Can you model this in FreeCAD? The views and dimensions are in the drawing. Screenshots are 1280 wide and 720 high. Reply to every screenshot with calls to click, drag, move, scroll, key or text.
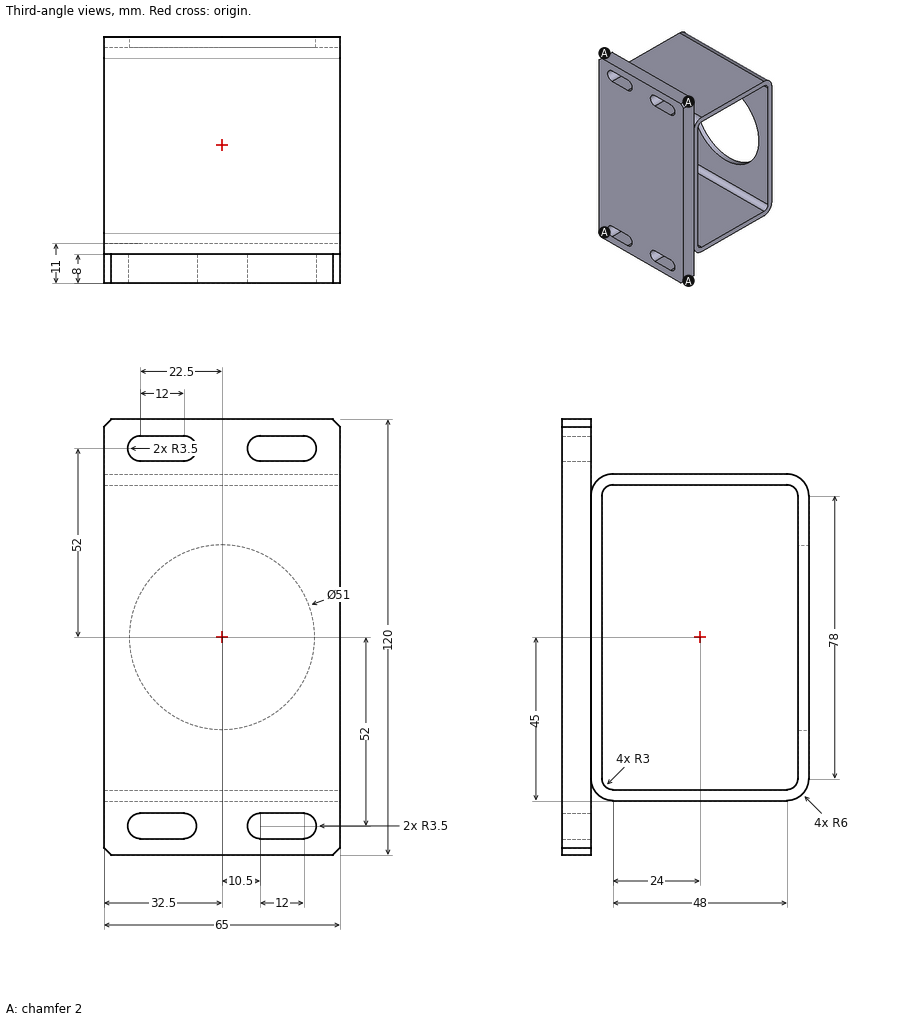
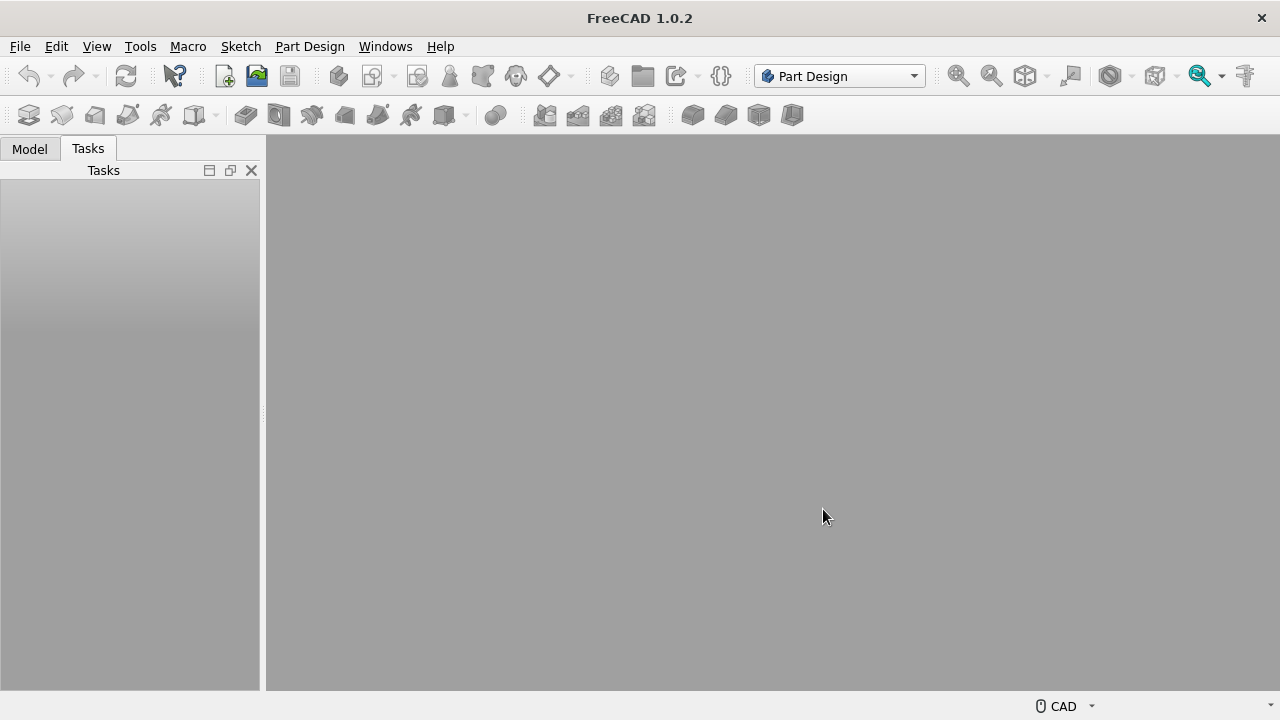
click(224, 76)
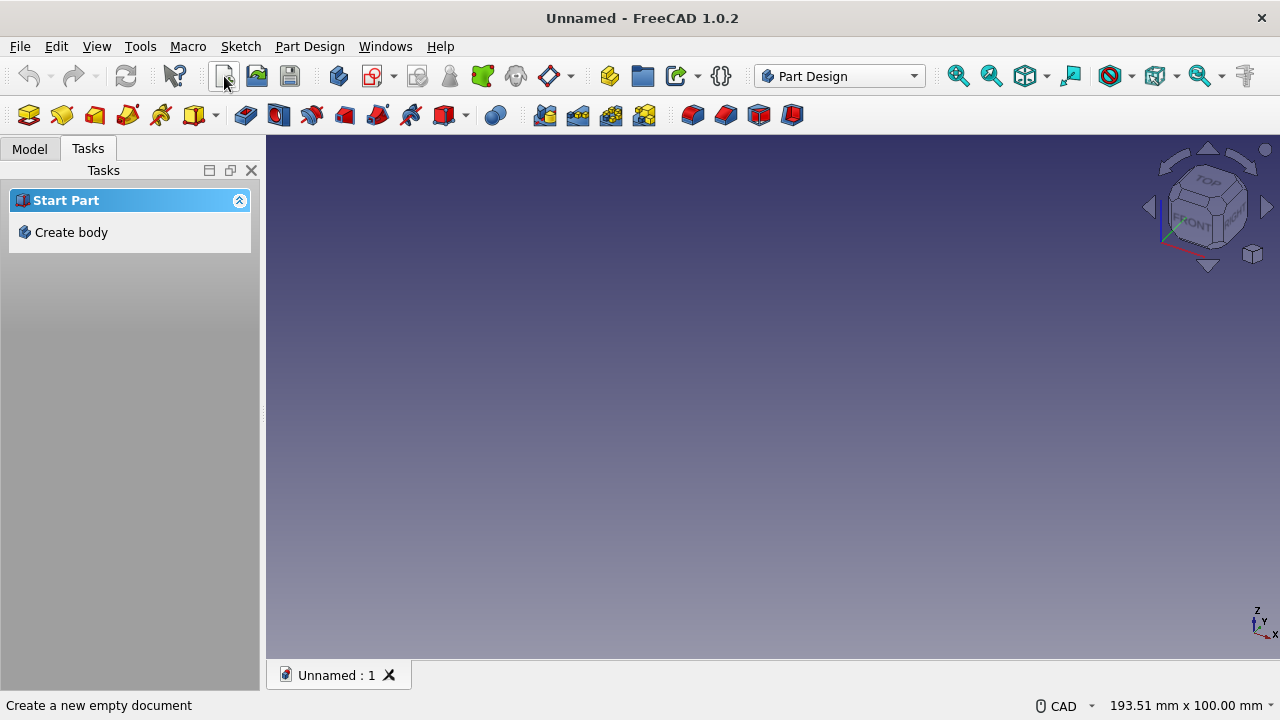
click(339, 76)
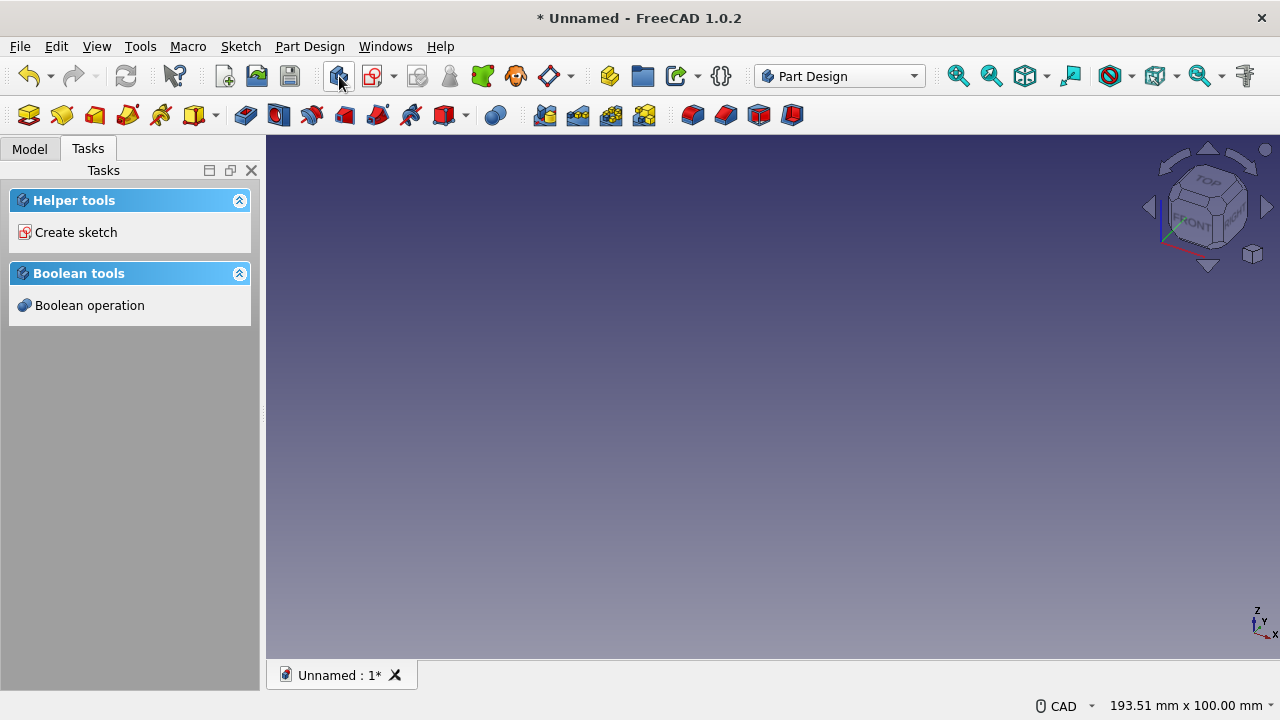
click(30, 148)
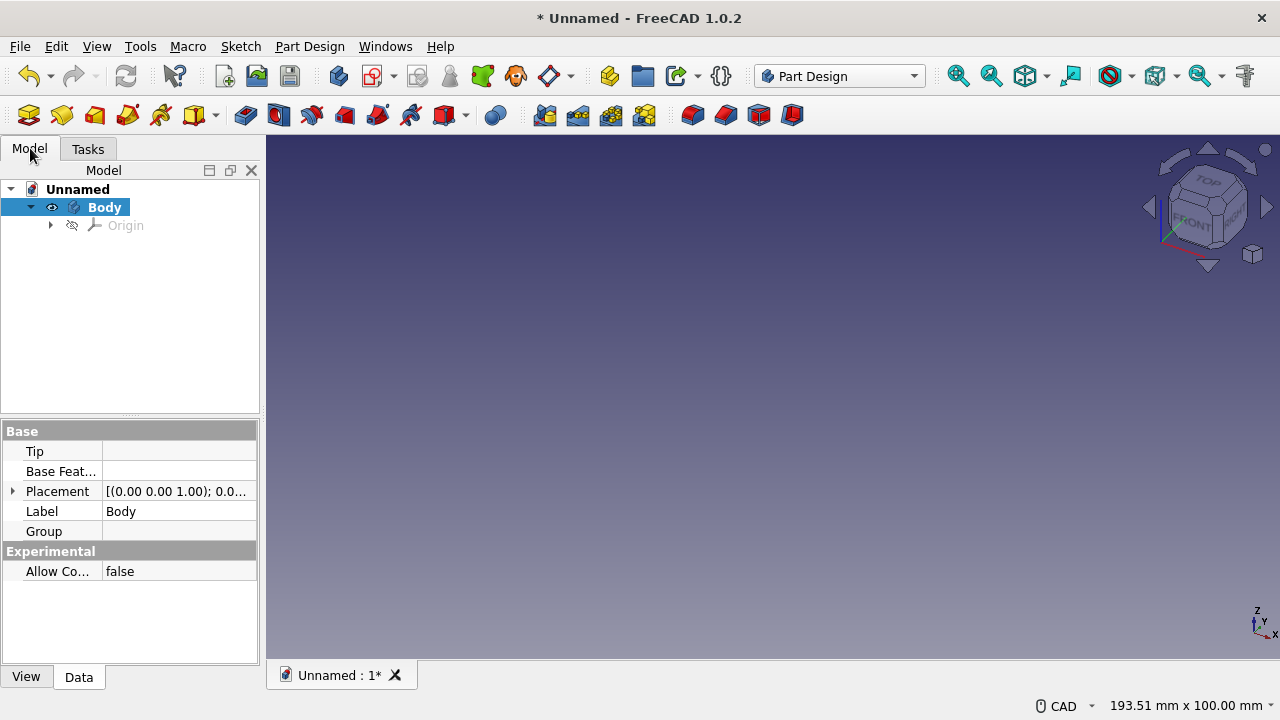
click(51, 225)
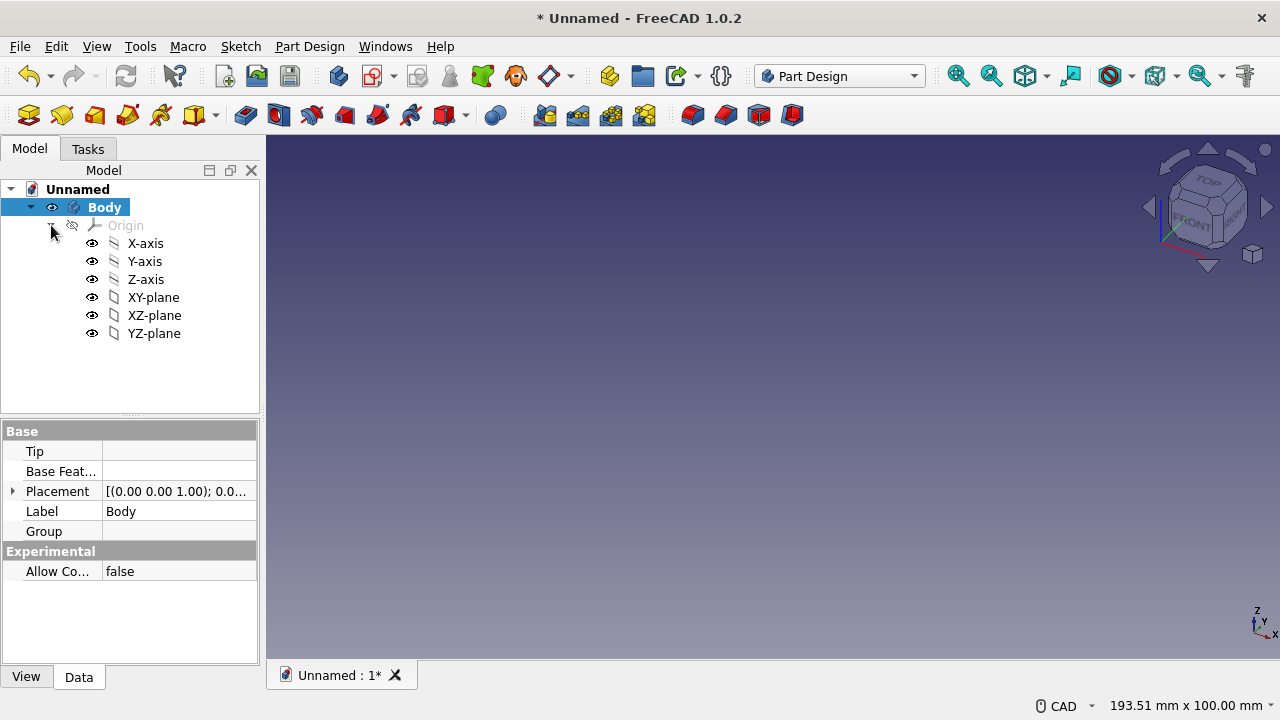
click(137, 333)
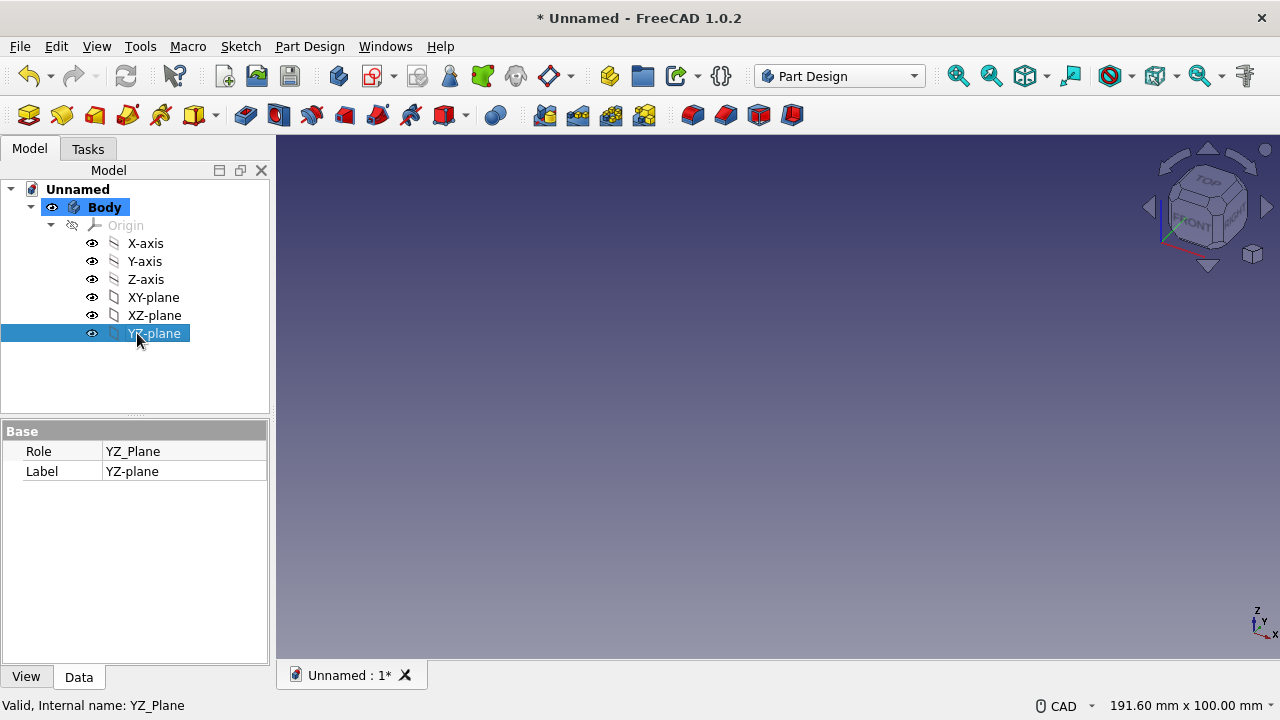
click(548, 76)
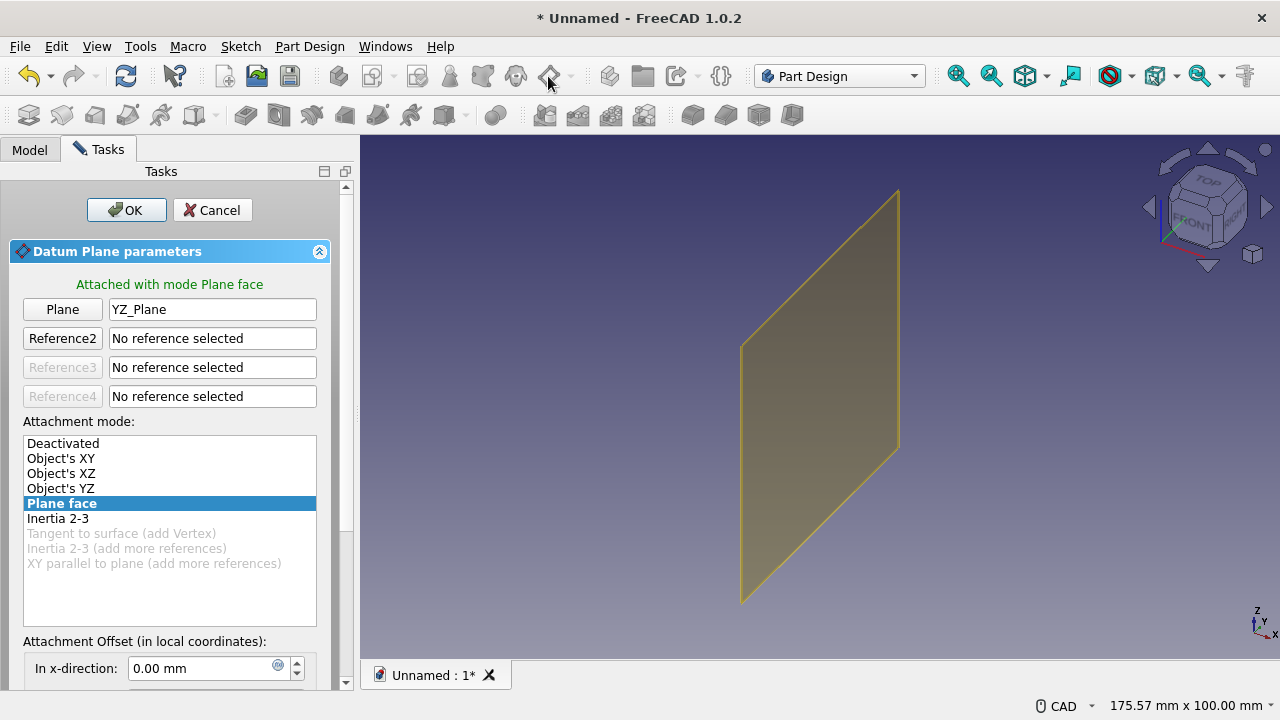
scroll(346, 436, down, 2)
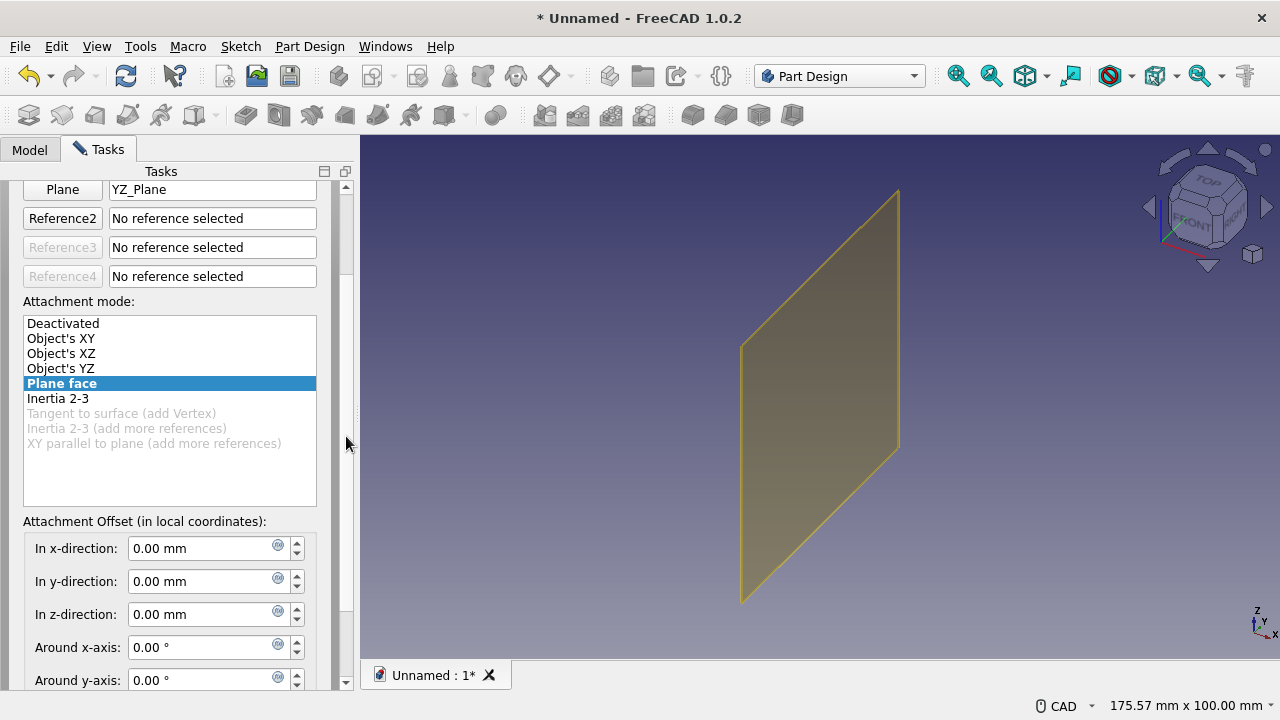
triple_click(210, 614)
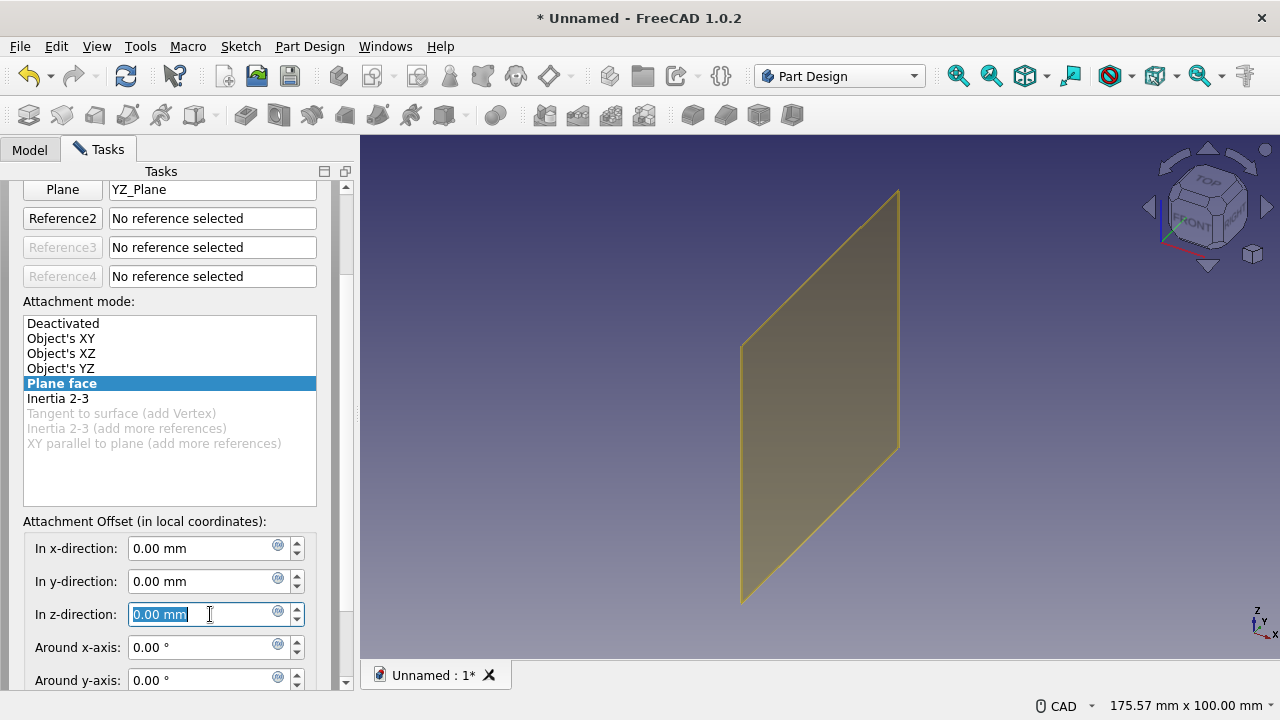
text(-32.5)
key(Tab)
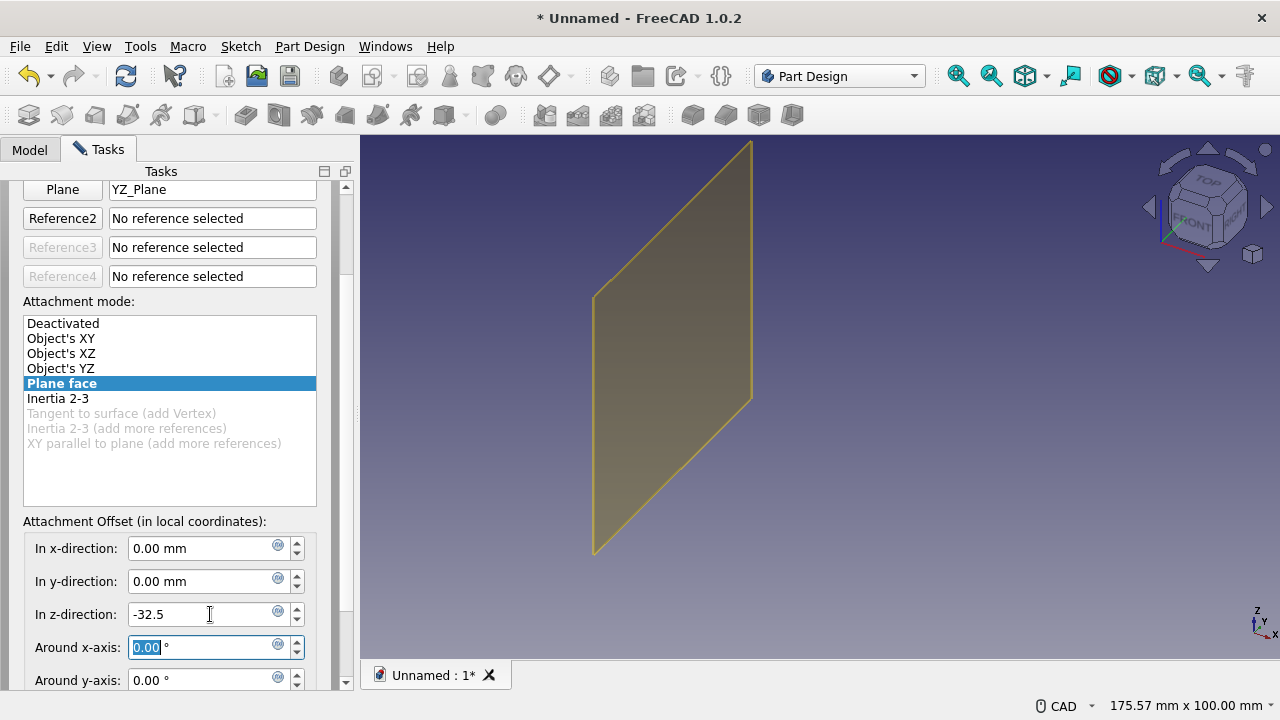
scroll(346, 436, up, 3)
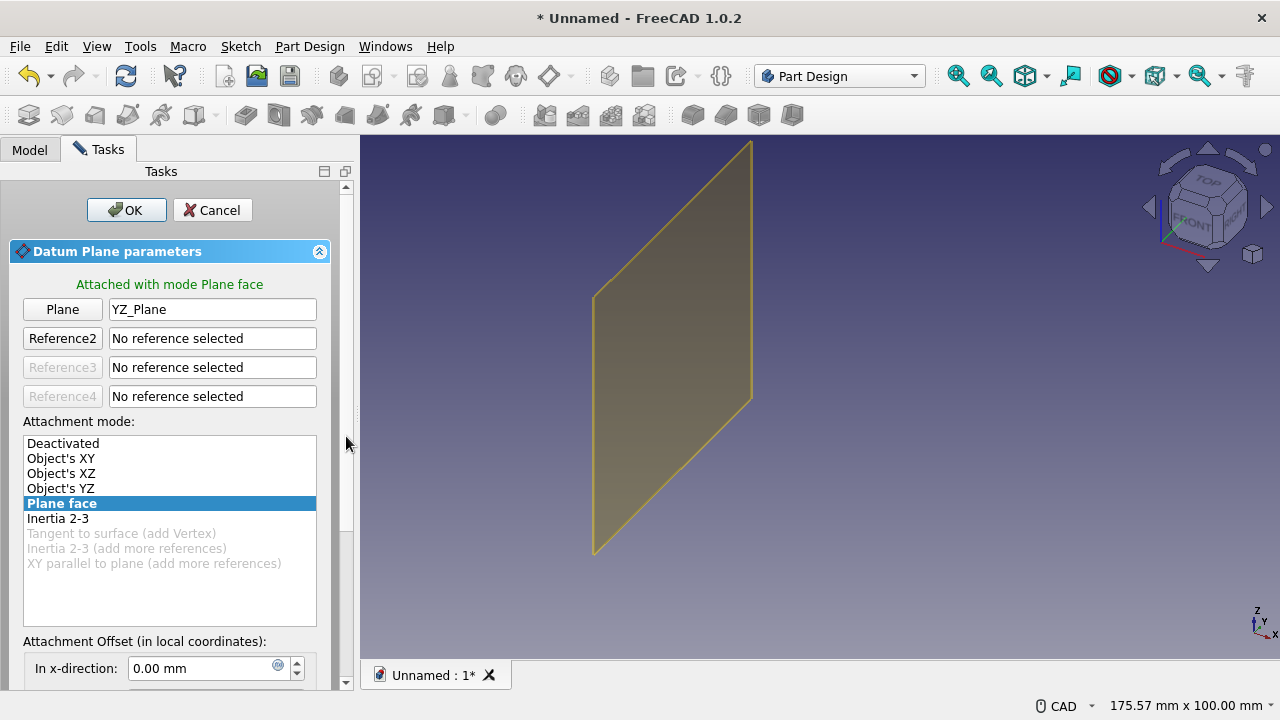
click(127, 210)